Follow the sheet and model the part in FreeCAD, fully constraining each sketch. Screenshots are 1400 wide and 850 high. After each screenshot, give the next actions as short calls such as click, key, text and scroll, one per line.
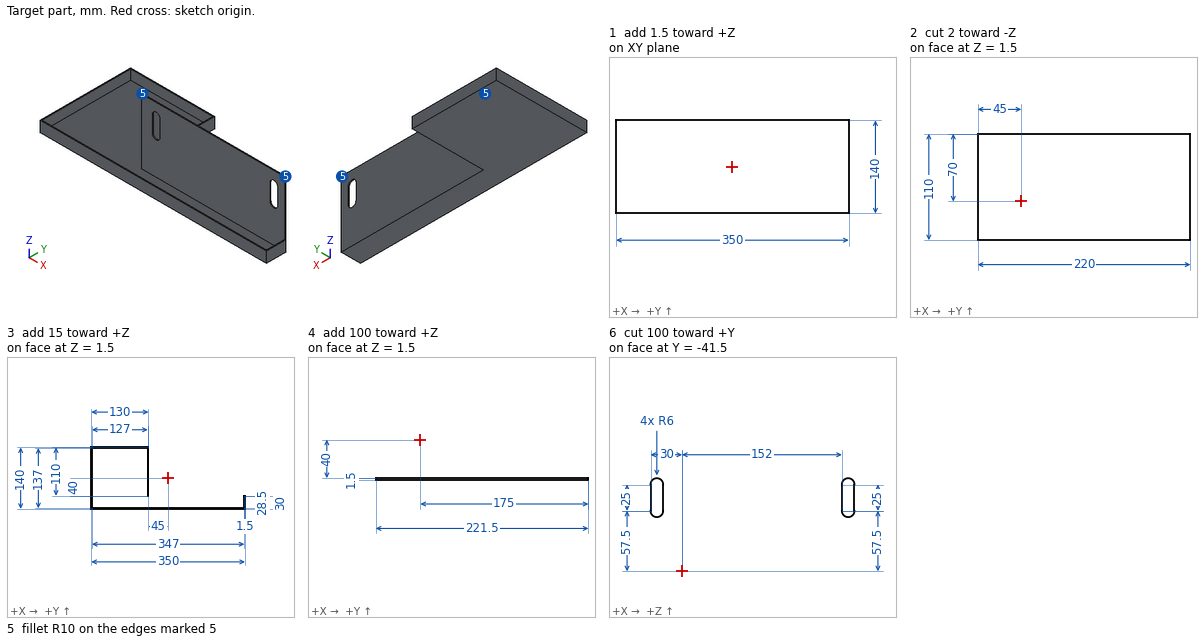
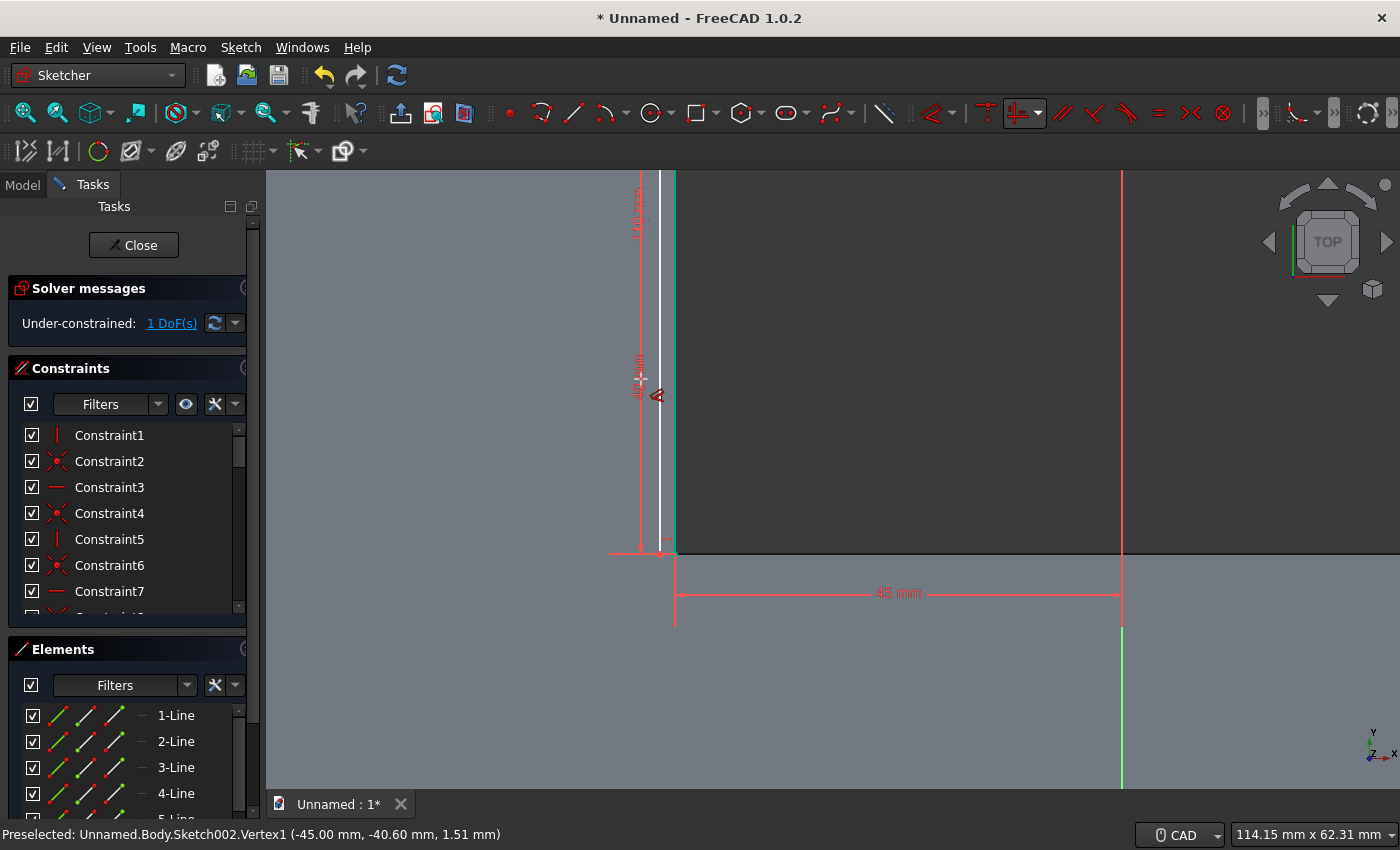
scroll(674, 561, down, 8)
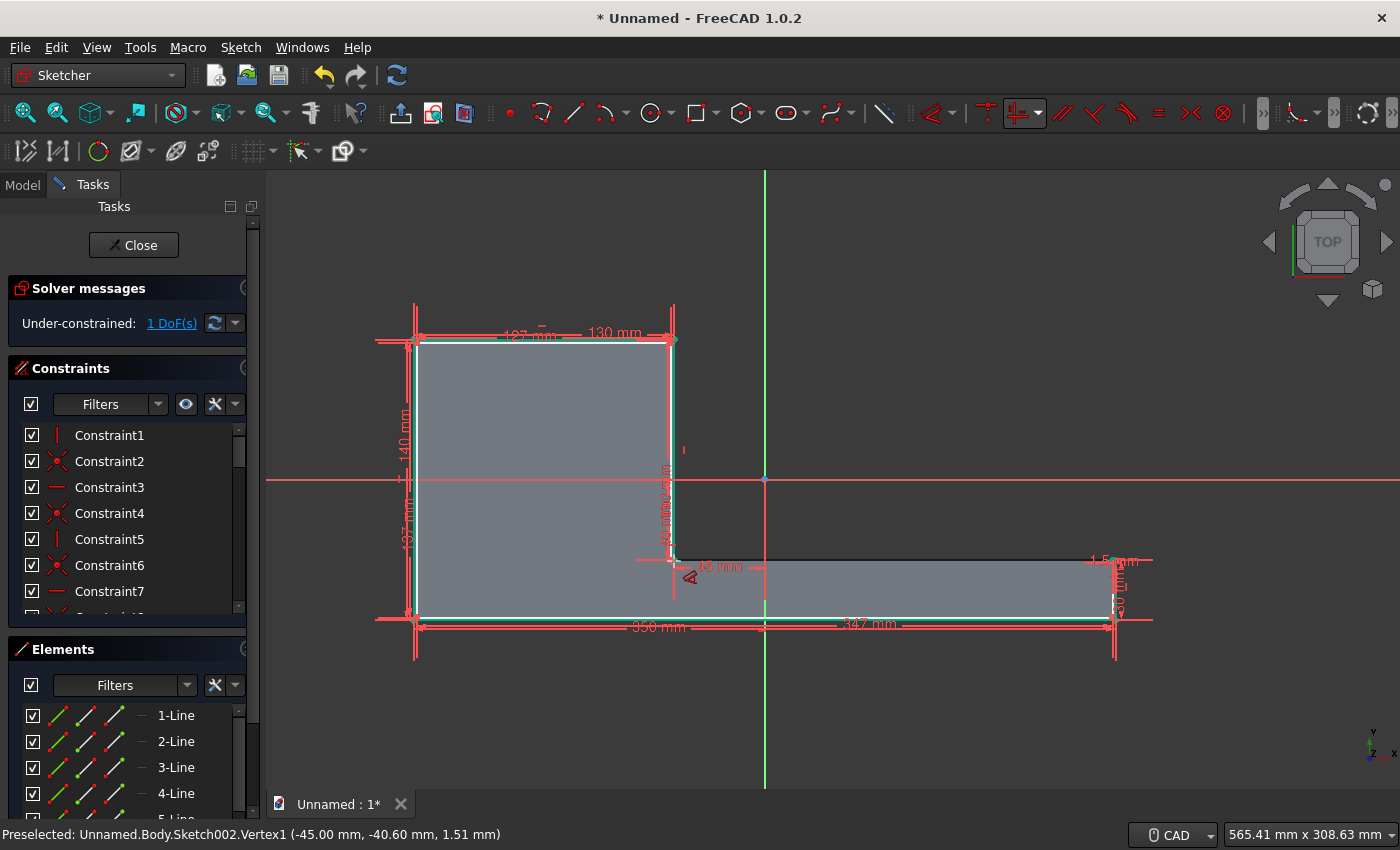
scroll(1113, 577, up, 8)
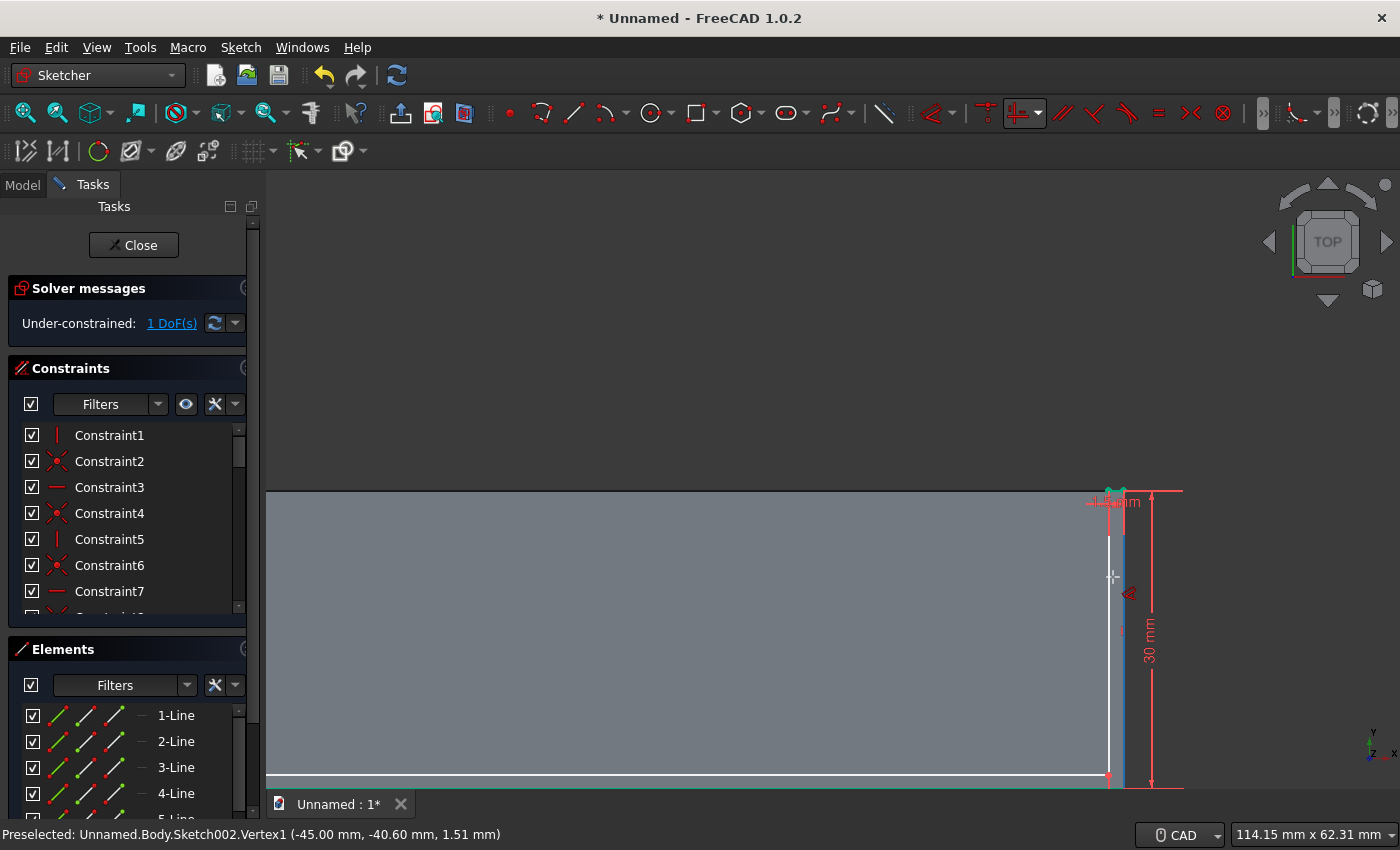
click(1109, 576)
click(1143, 564)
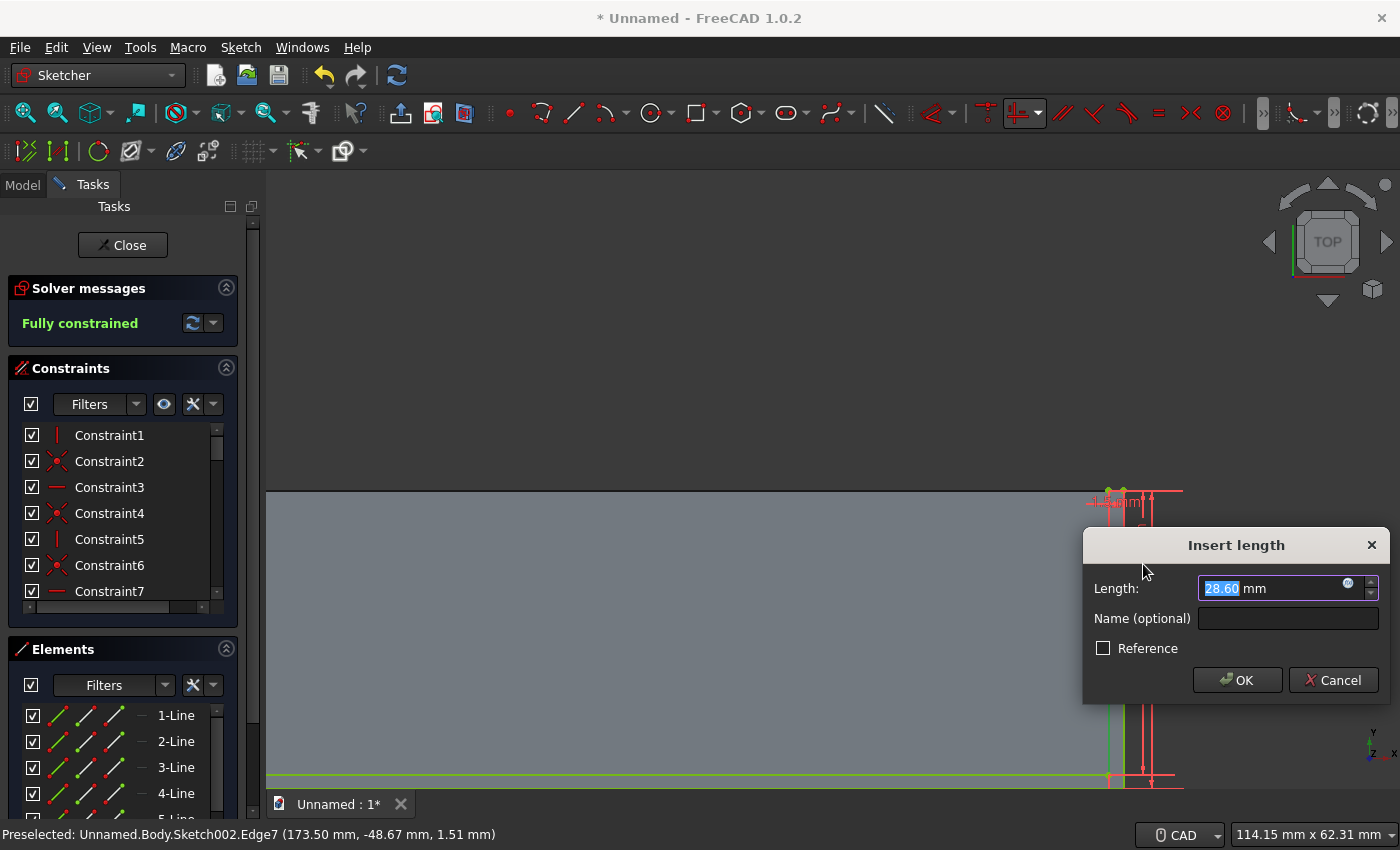
text(28.5)
key(Return)
key(Escape)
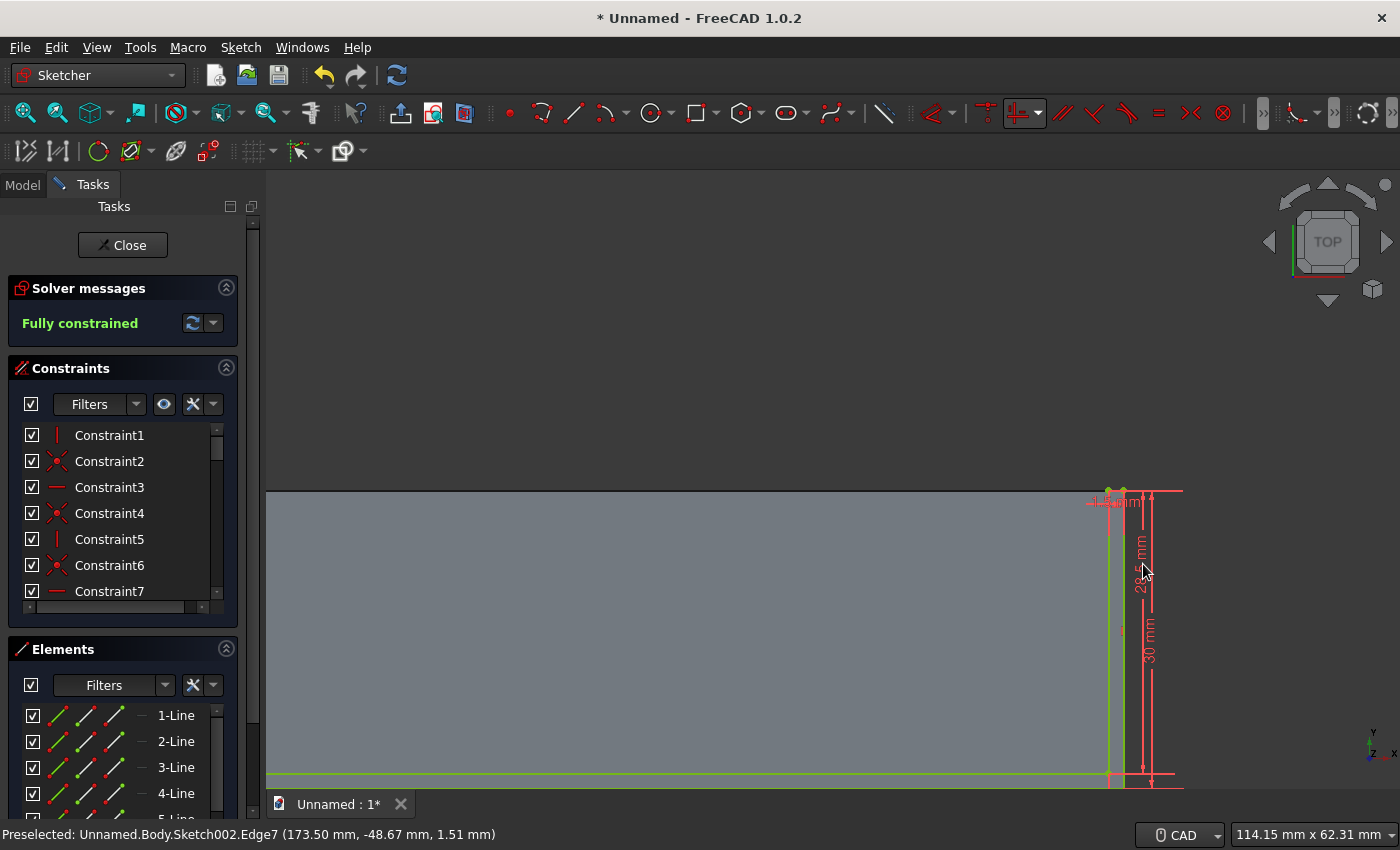
click(123, 245)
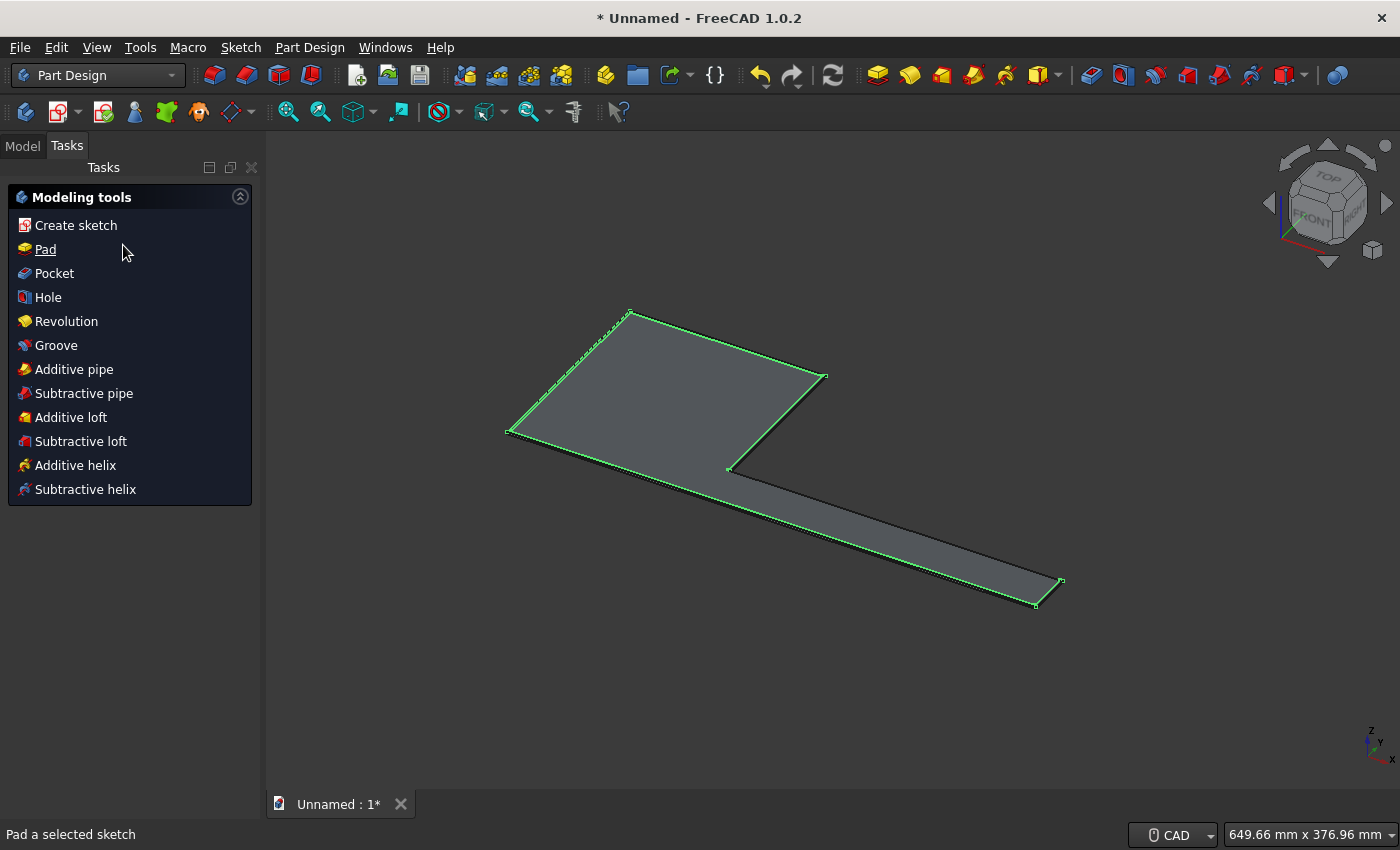
click(878, 76)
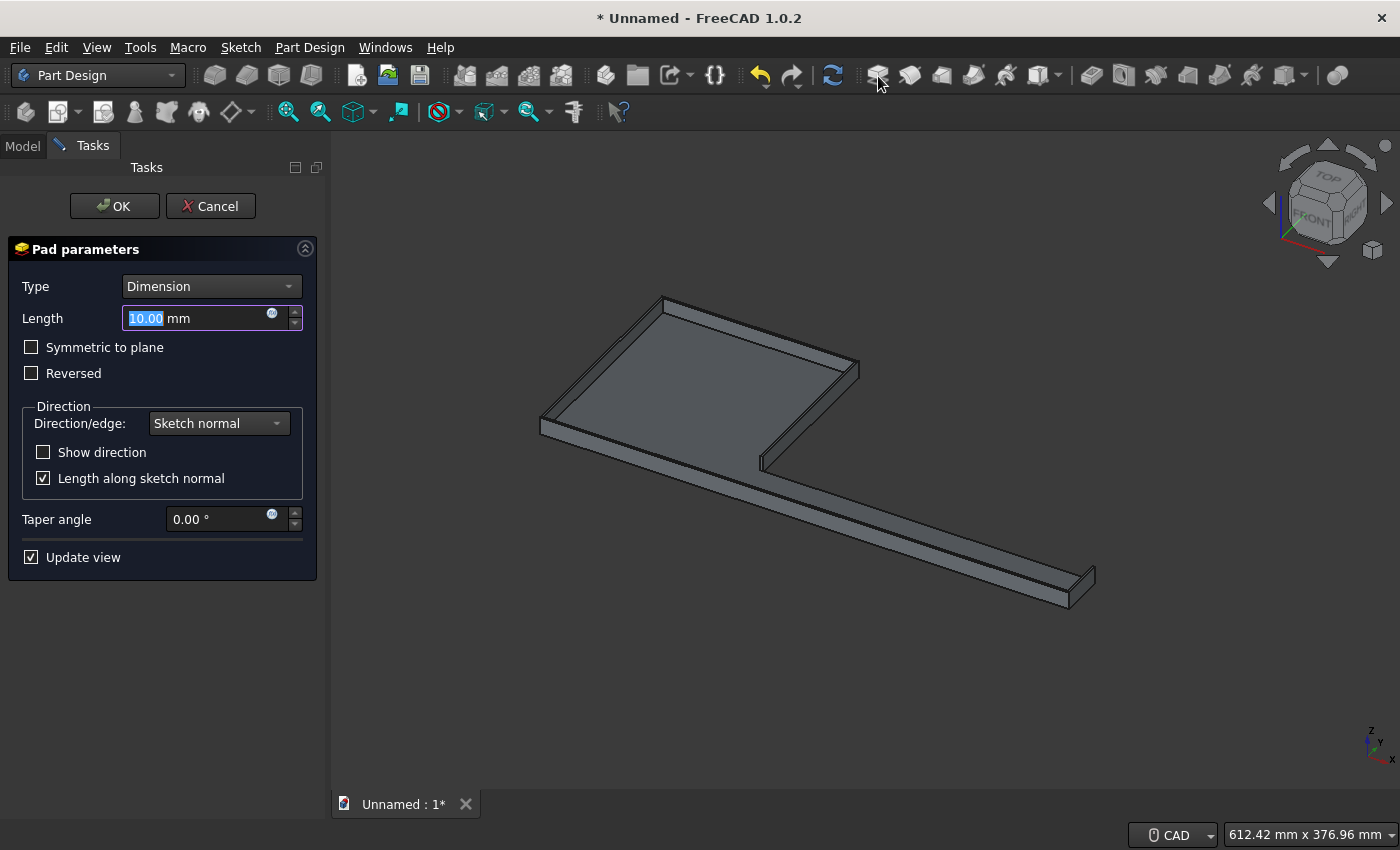
text(15)
key(Tab)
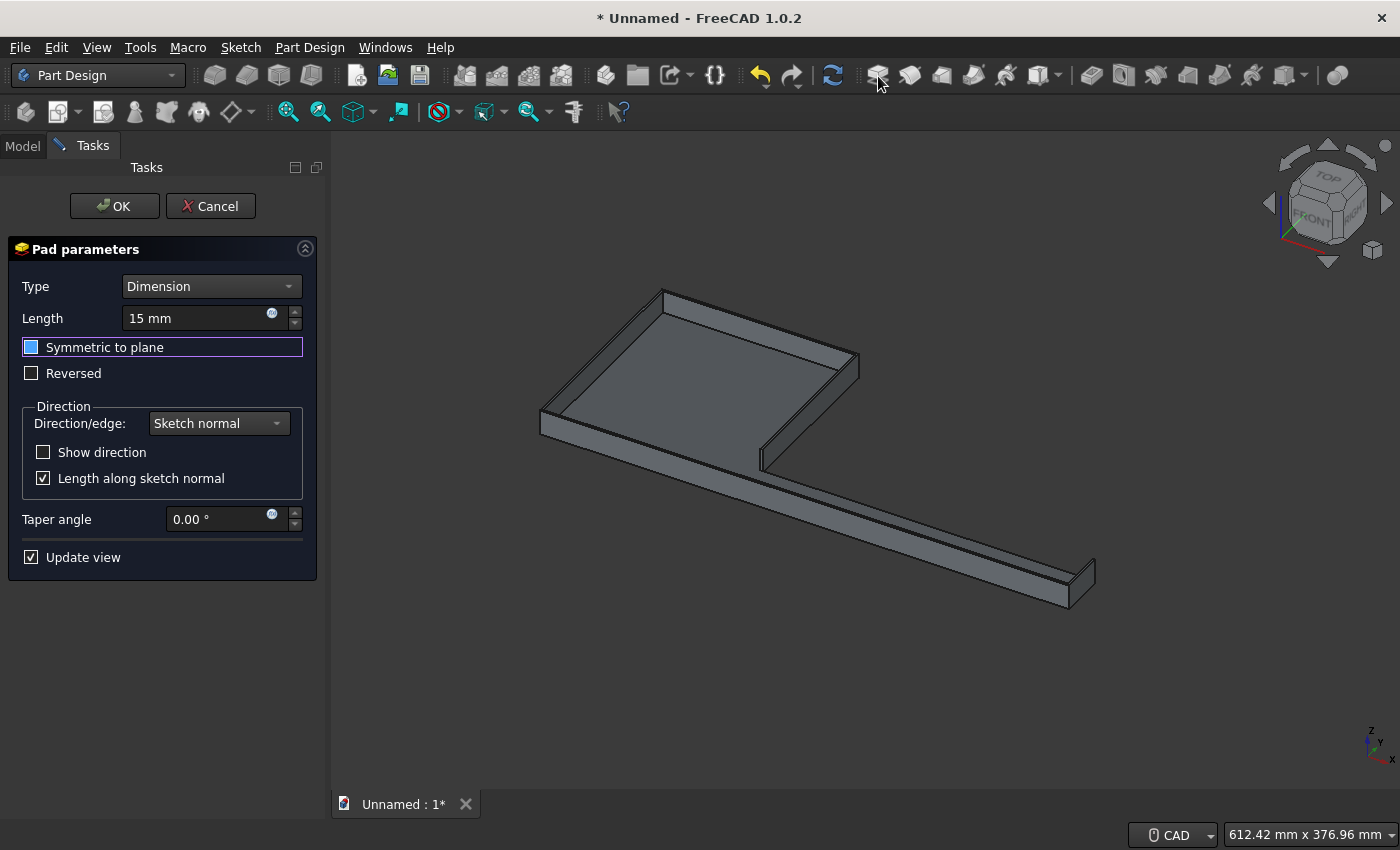
click(115, 206)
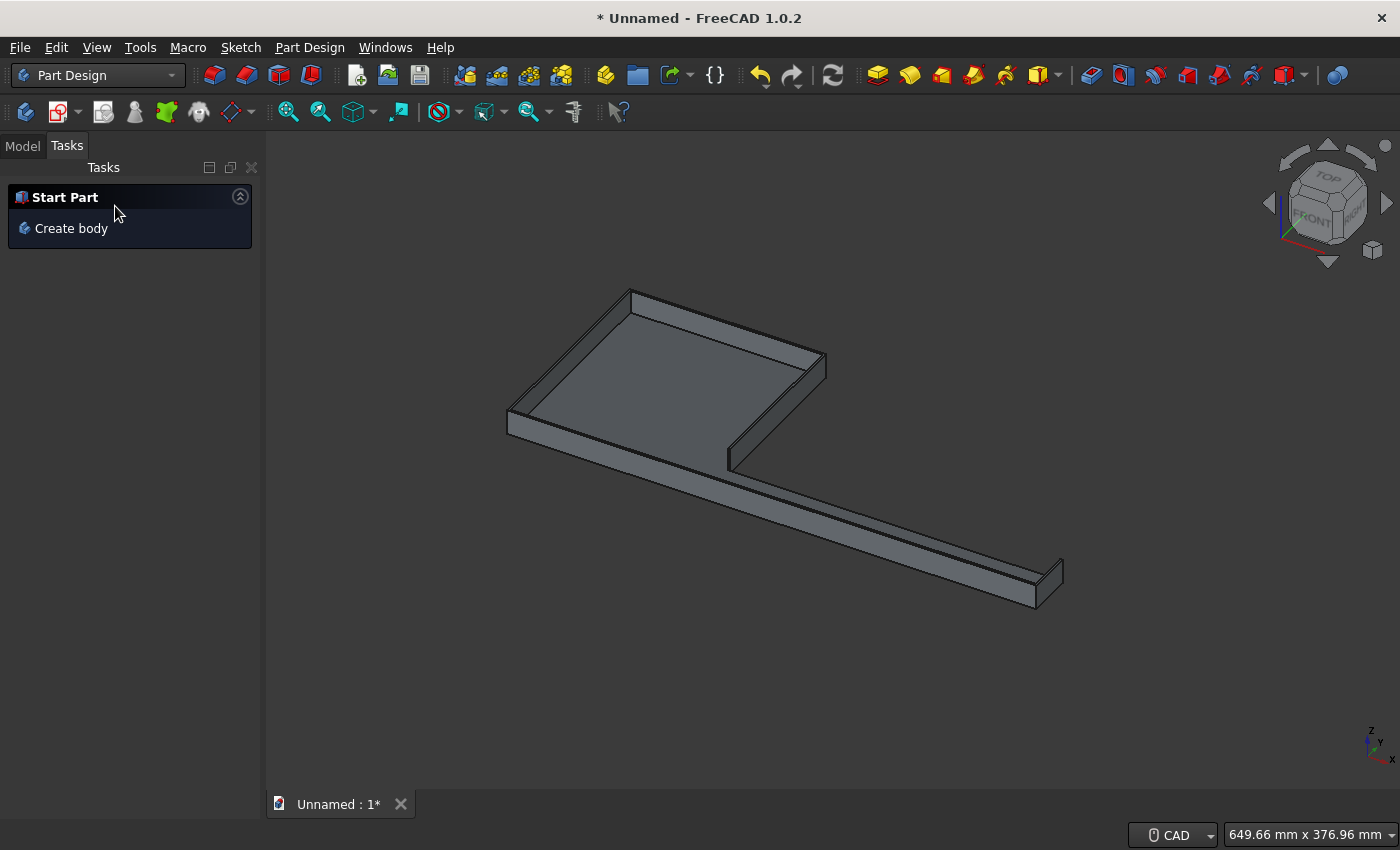
click(683, 408)